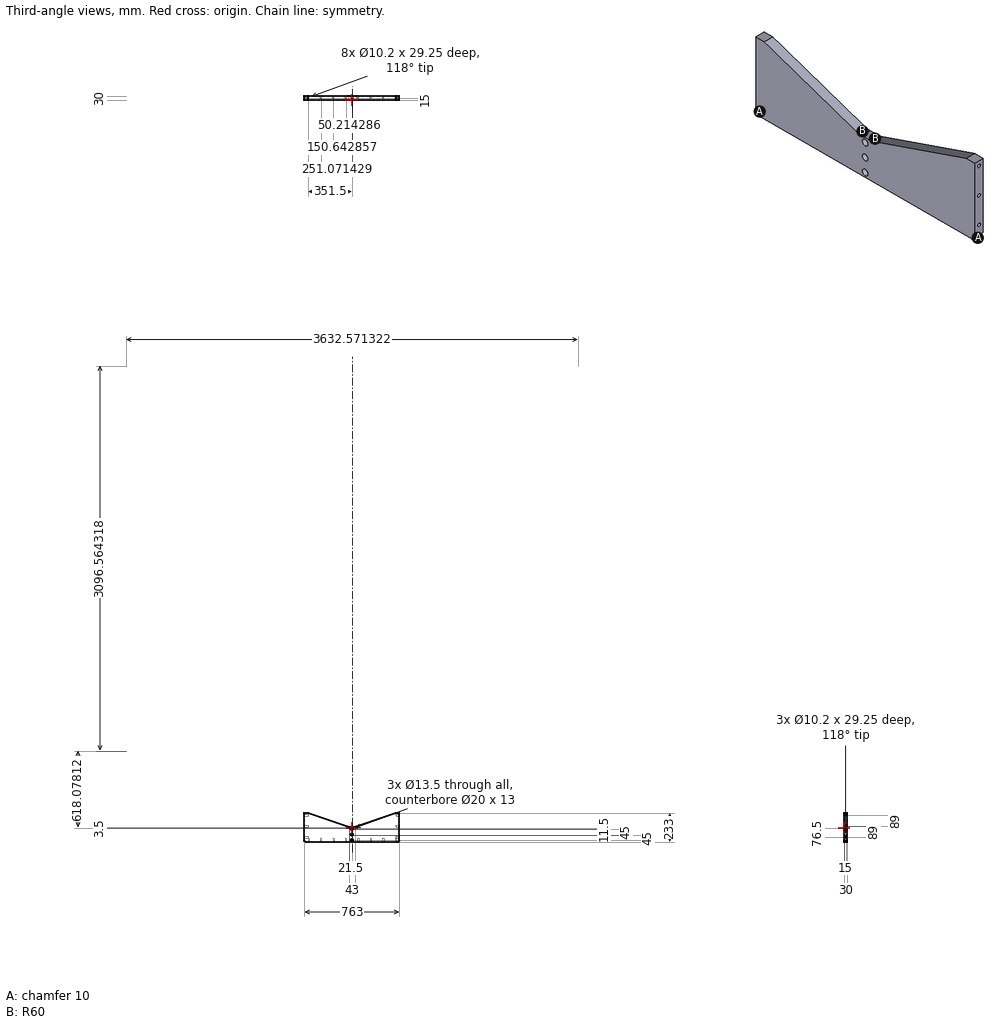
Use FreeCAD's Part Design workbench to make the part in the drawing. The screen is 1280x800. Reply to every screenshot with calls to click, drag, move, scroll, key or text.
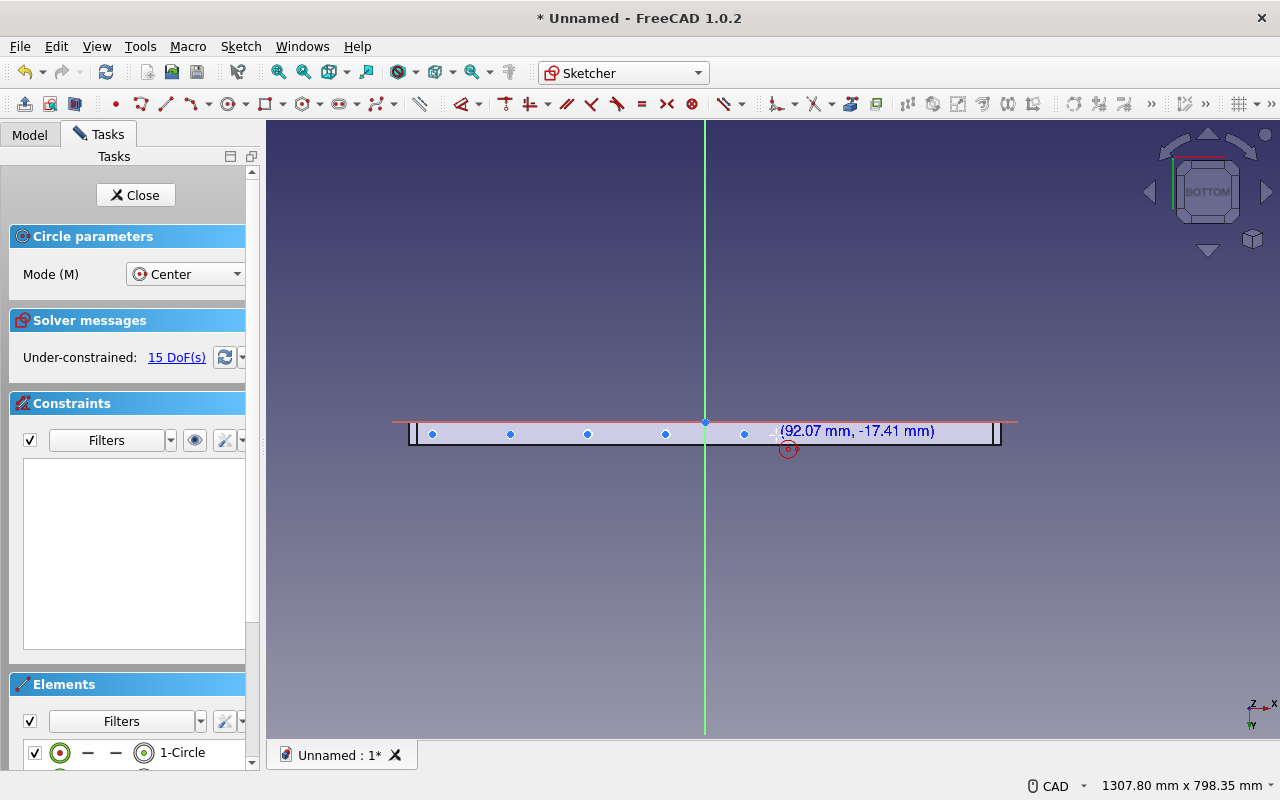
scroll(822, 434, up, 2)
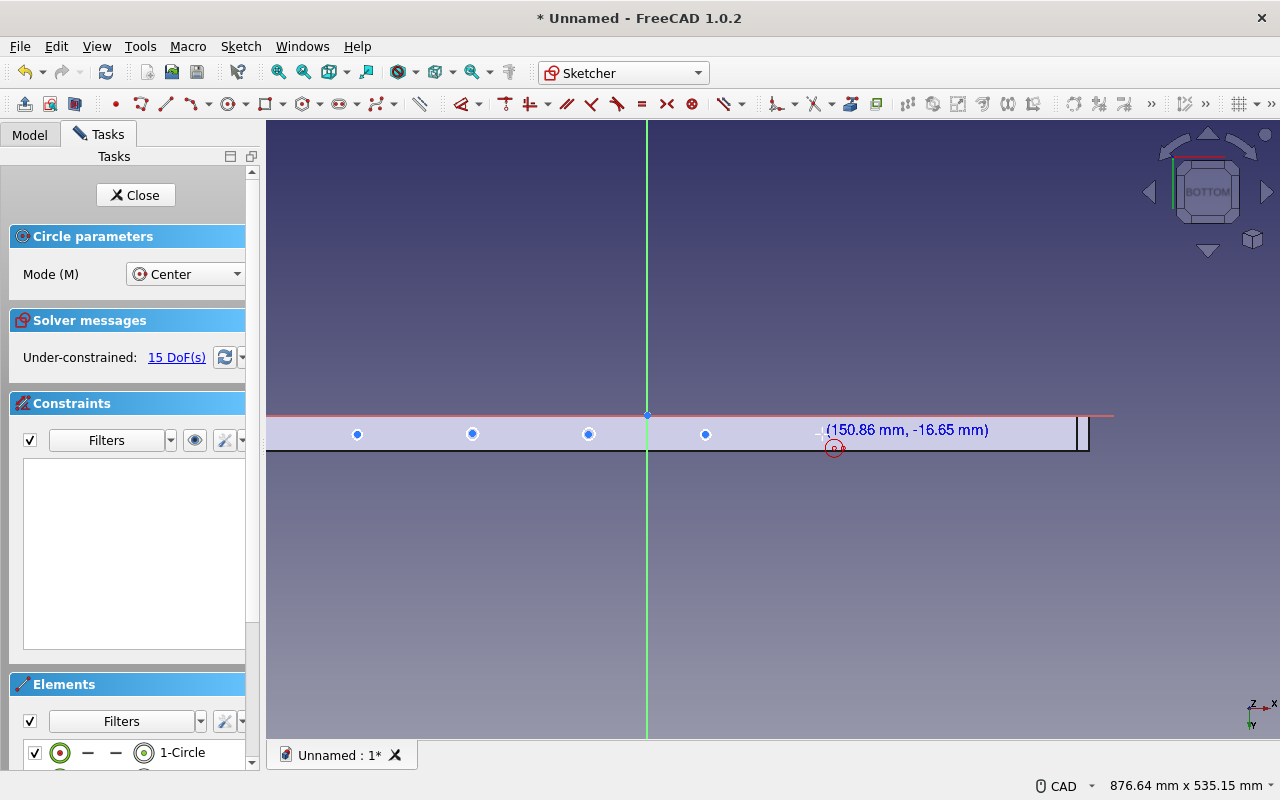
click(821, 433)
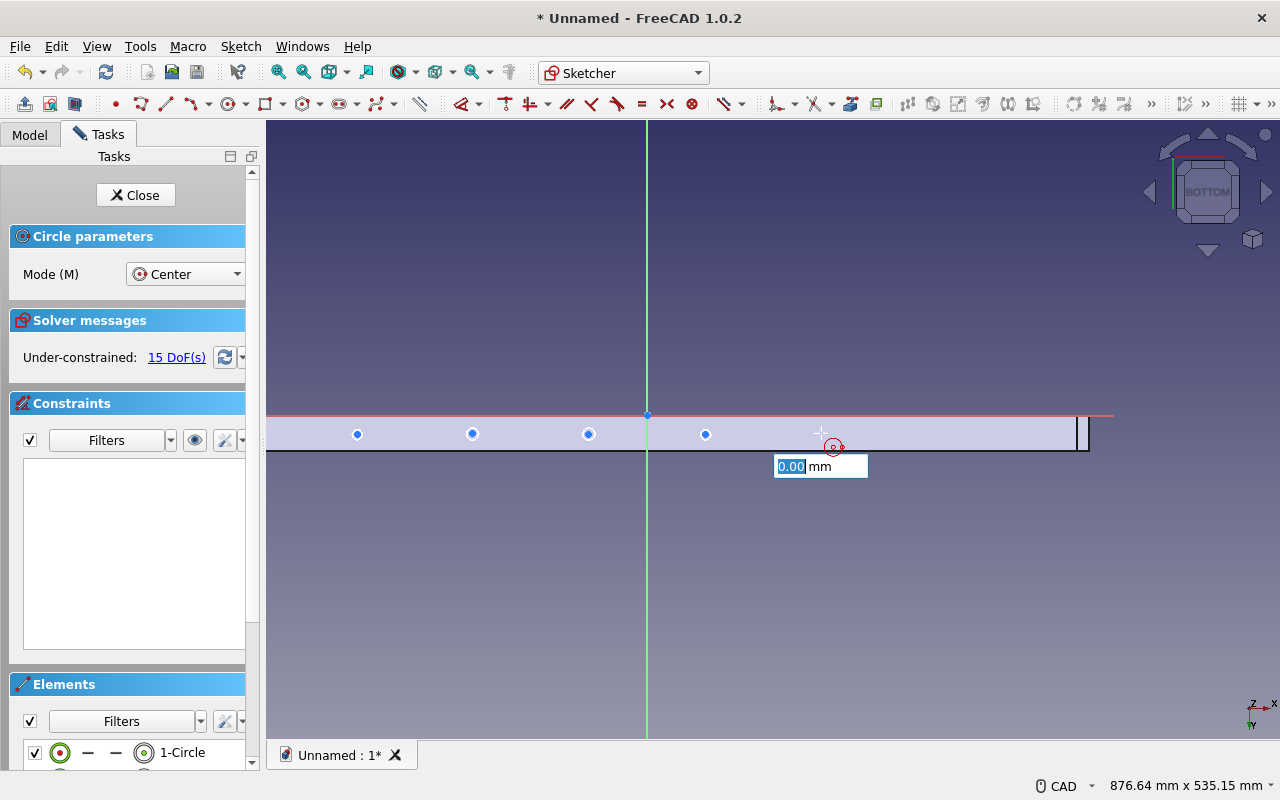
scroll(826, 438, up, 5)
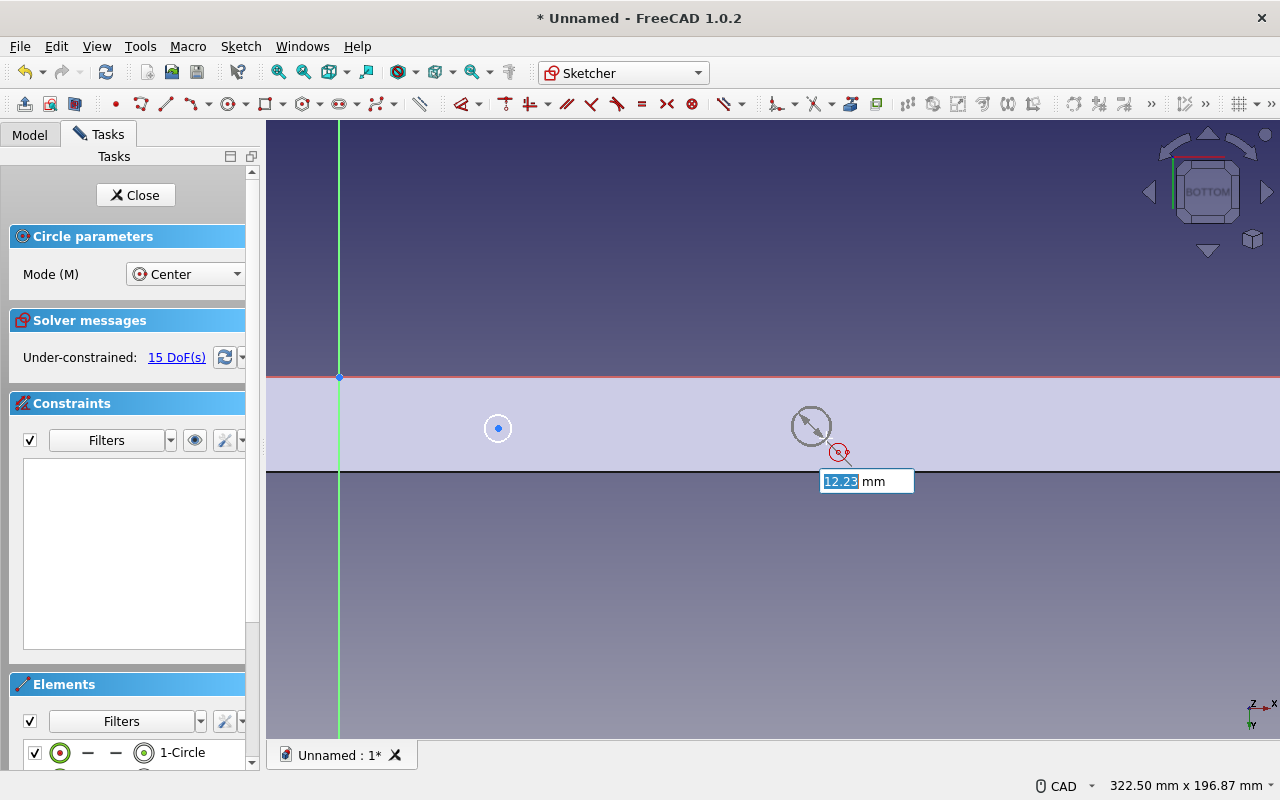
click(824, 436)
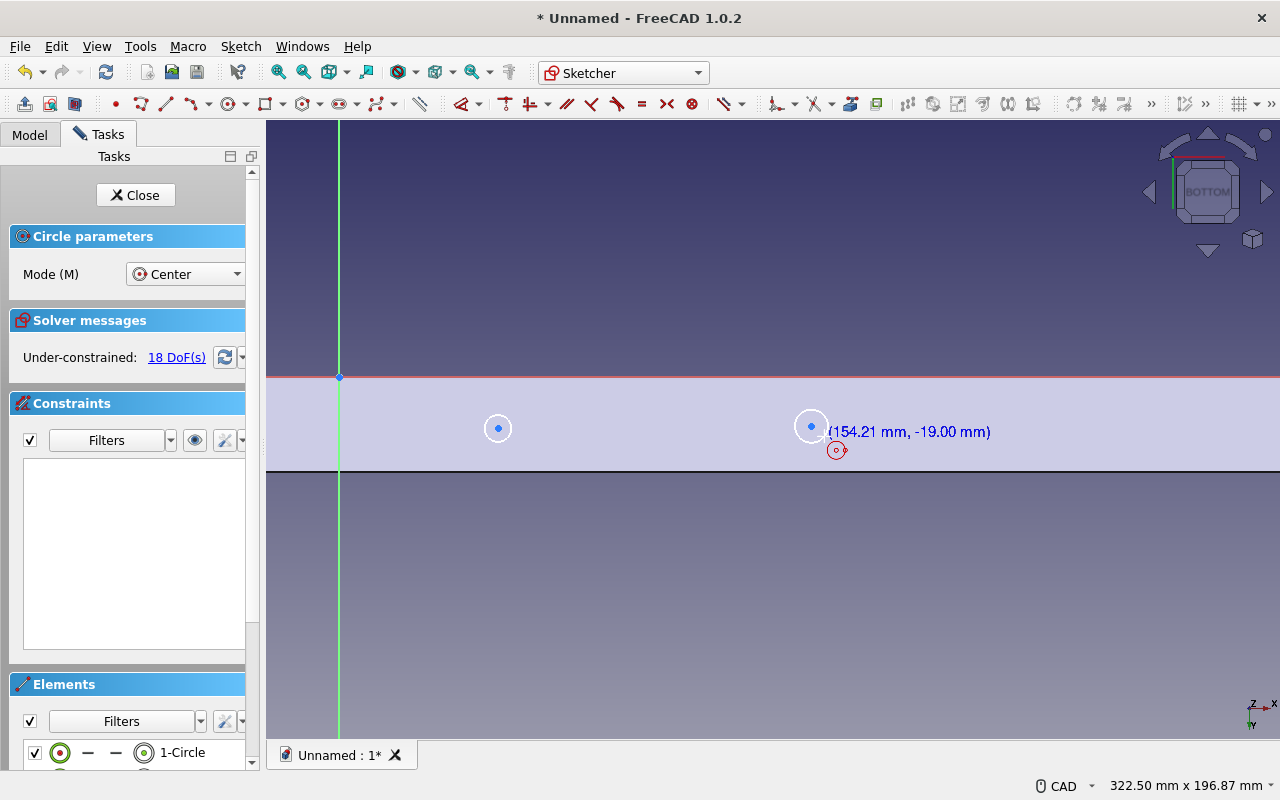
scroll(824, 436, down, 7)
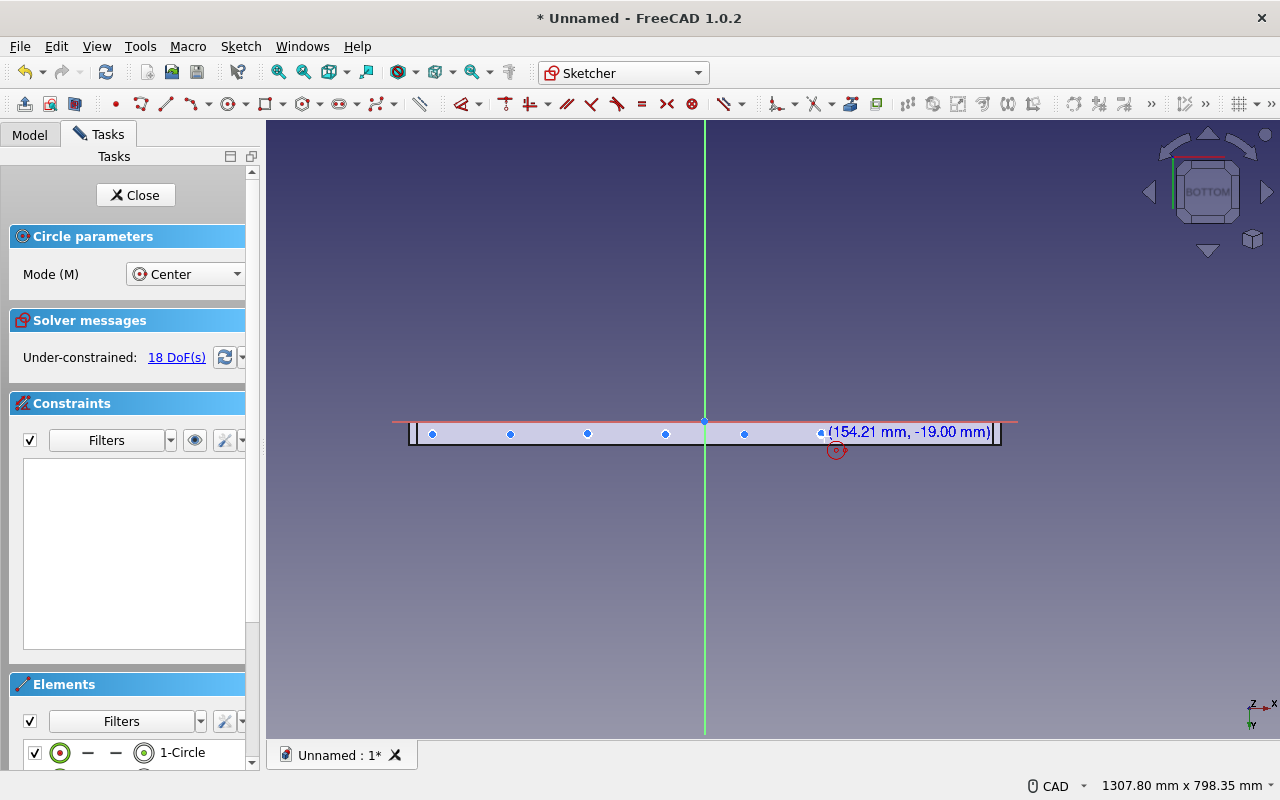
scroll(900, 434, up, 9)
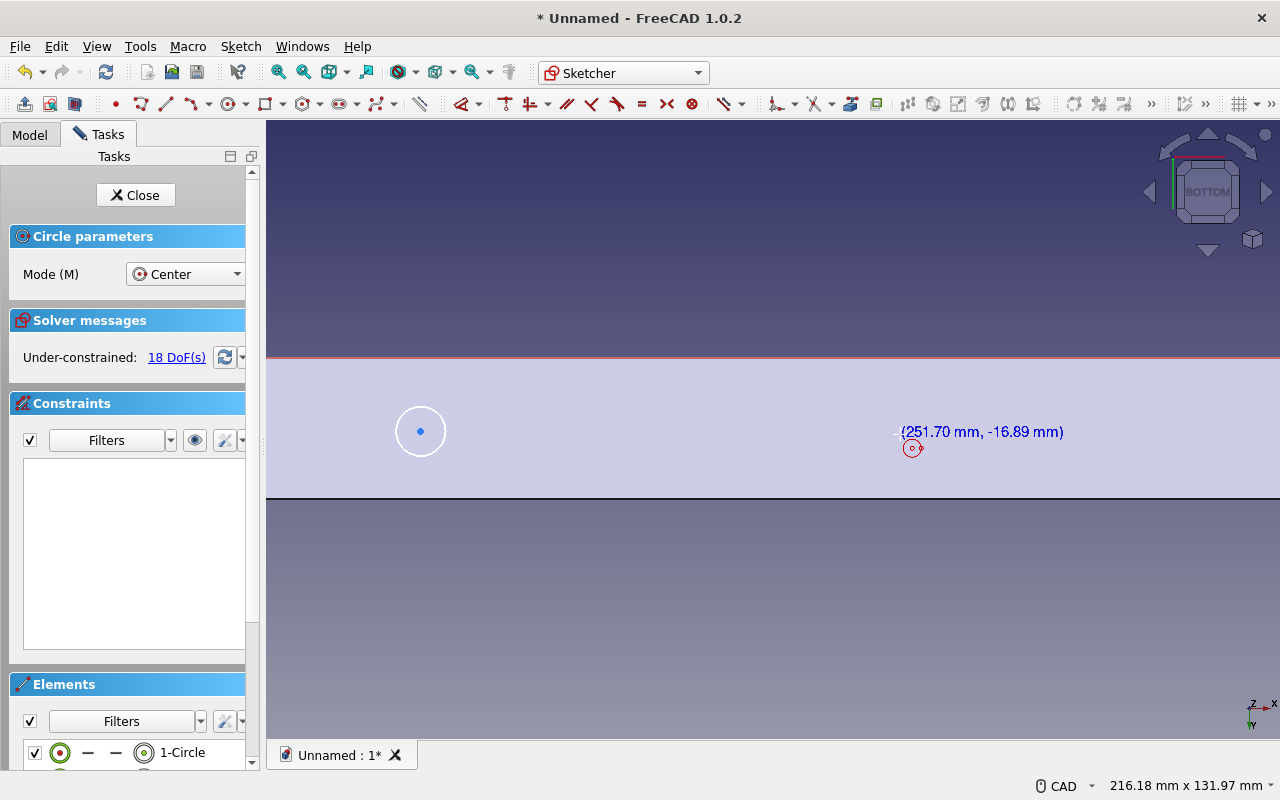
scroll(900, 434, down, 9)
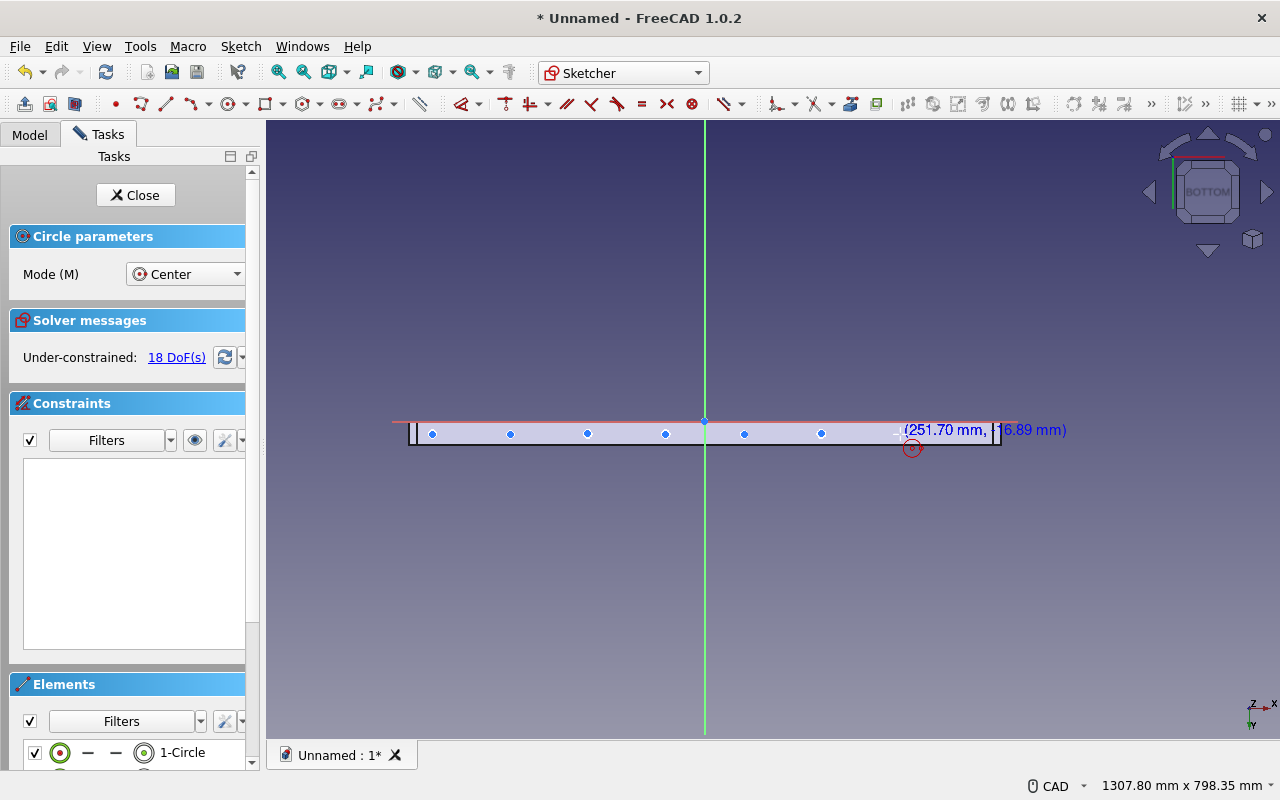
scroll(900, 434, up, 2)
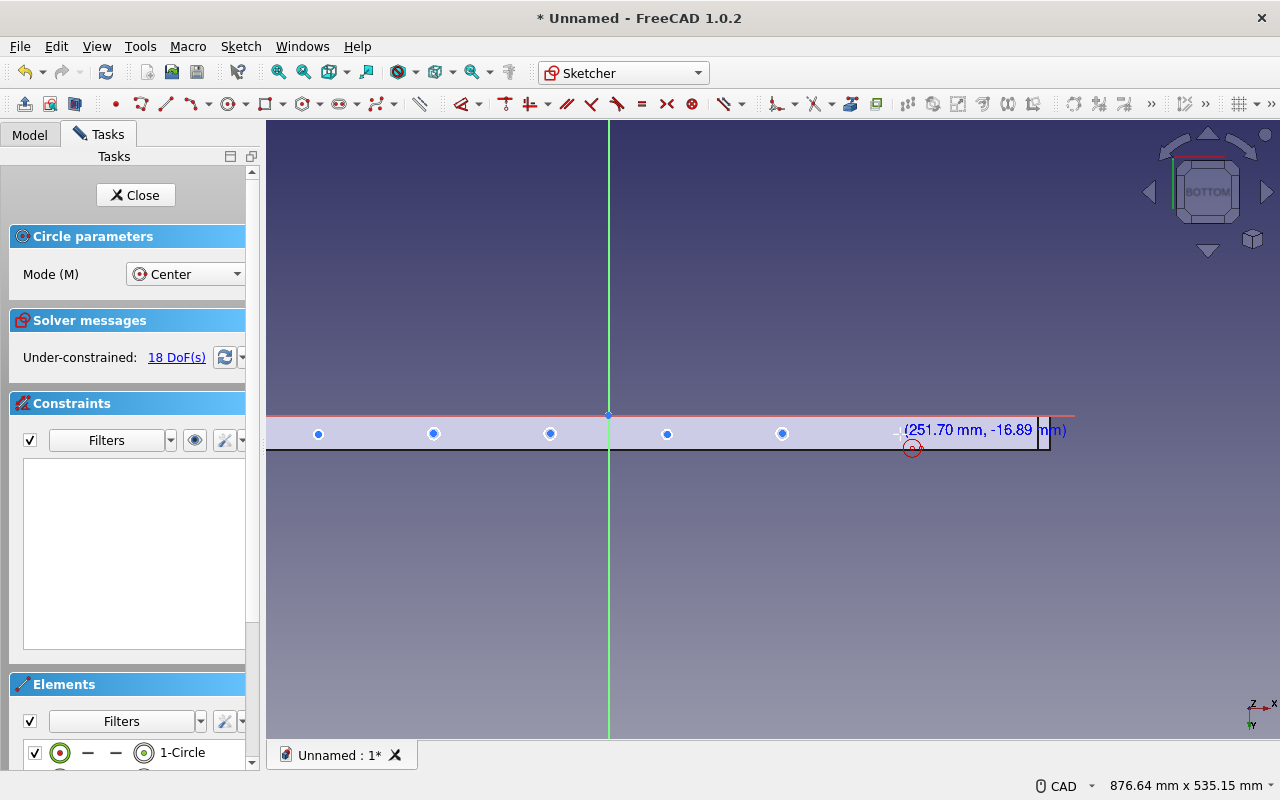
click(899, 433)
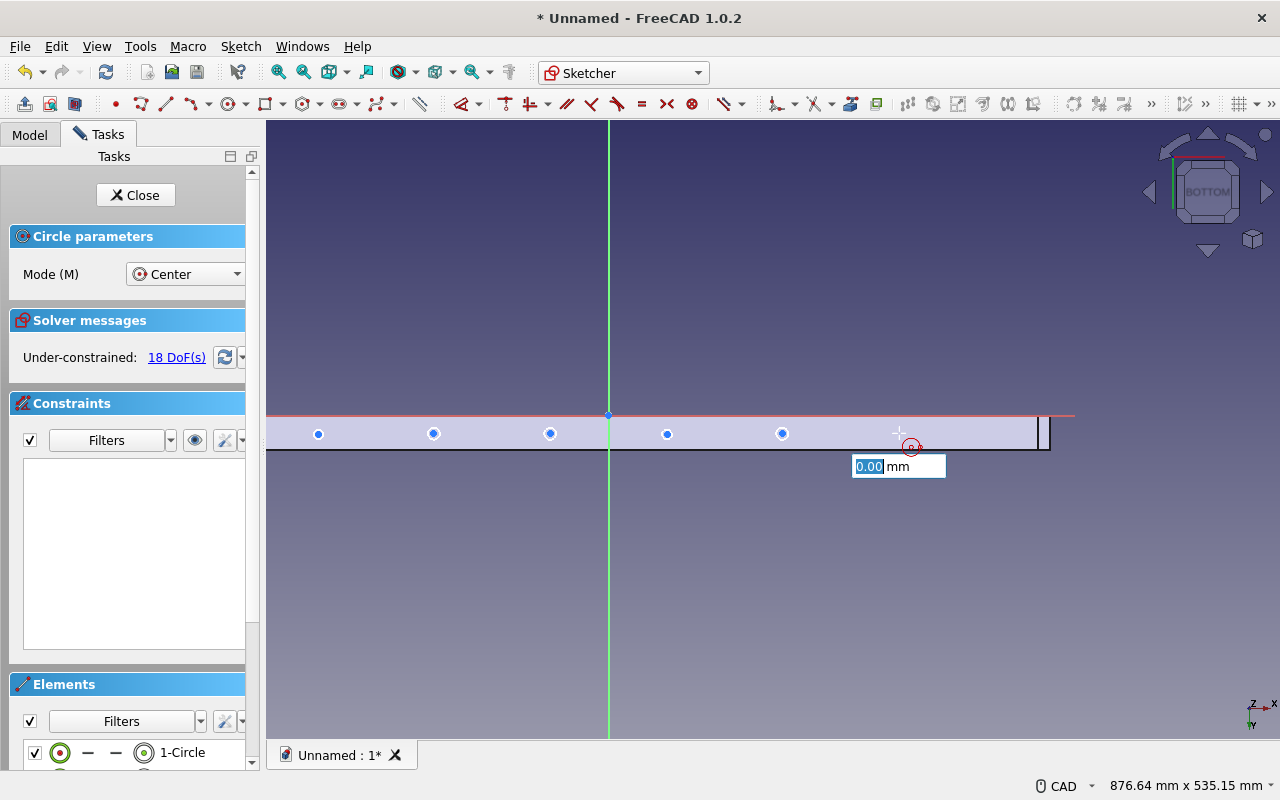
scroll(903, 437, up, 5)